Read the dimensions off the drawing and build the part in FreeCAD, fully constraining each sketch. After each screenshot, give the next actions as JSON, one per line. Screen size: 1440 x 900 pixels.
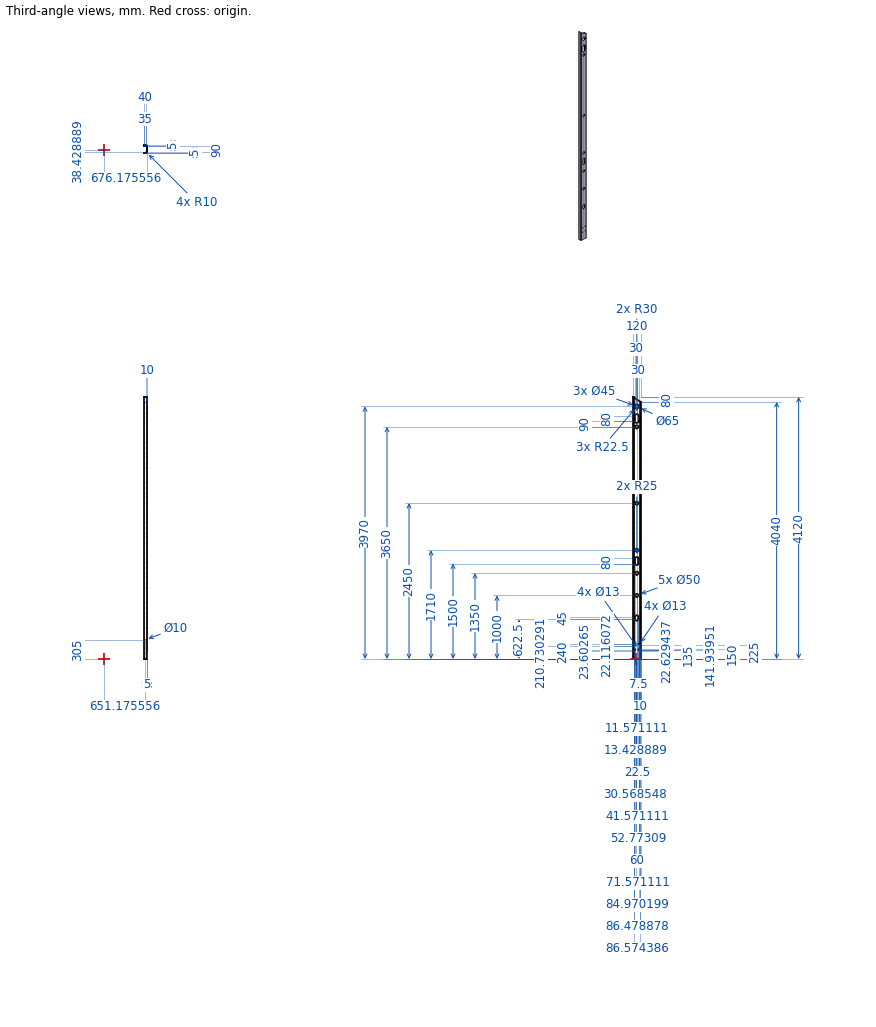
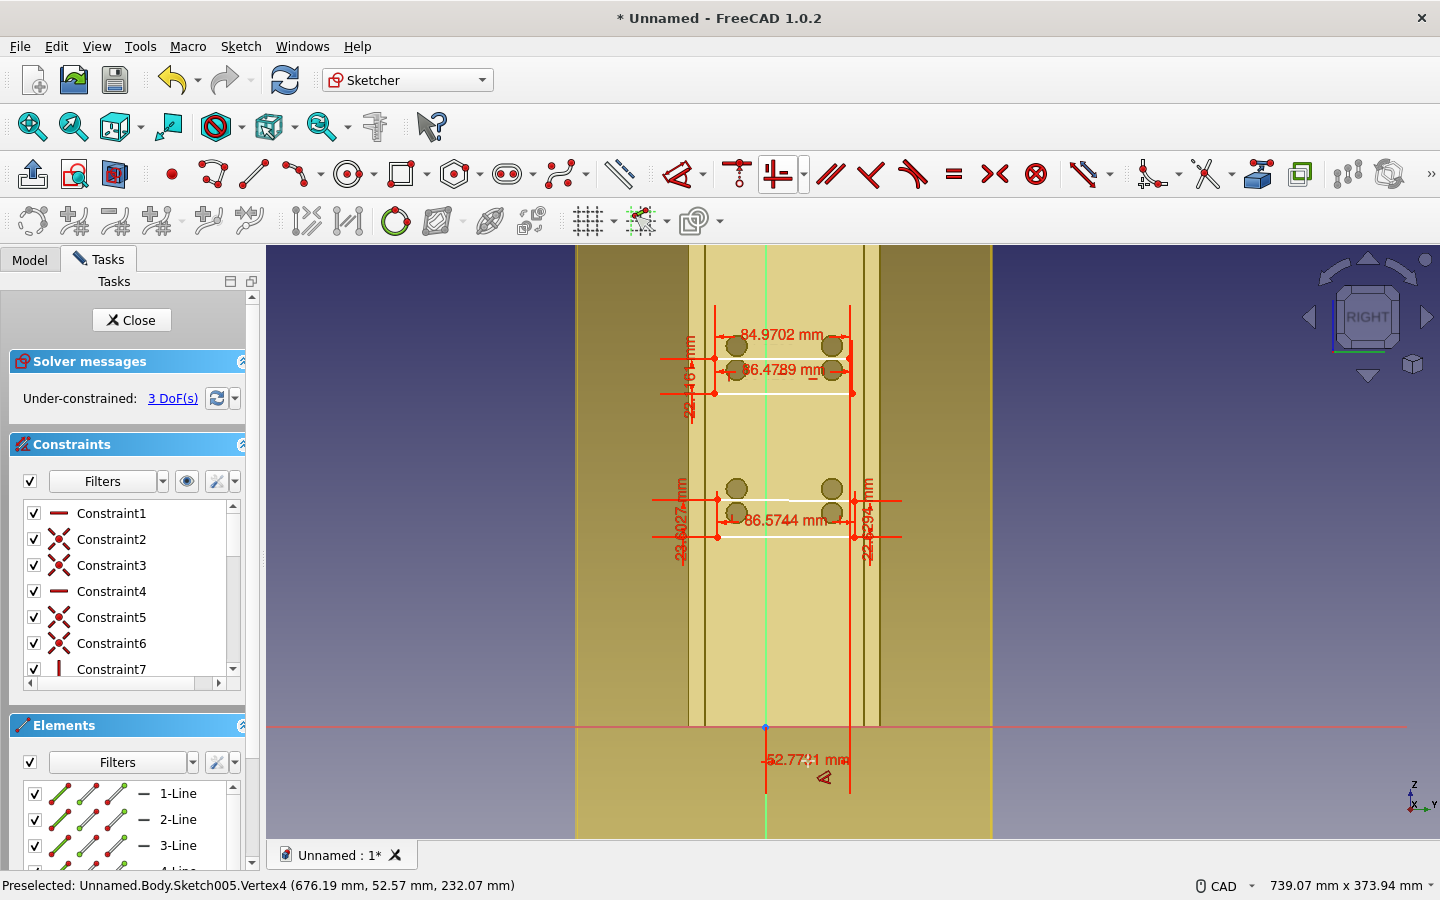
{"action": "left_click", "coordinate": [717, 537]}
{"action": "left_click", "coordinate": [730, 761]}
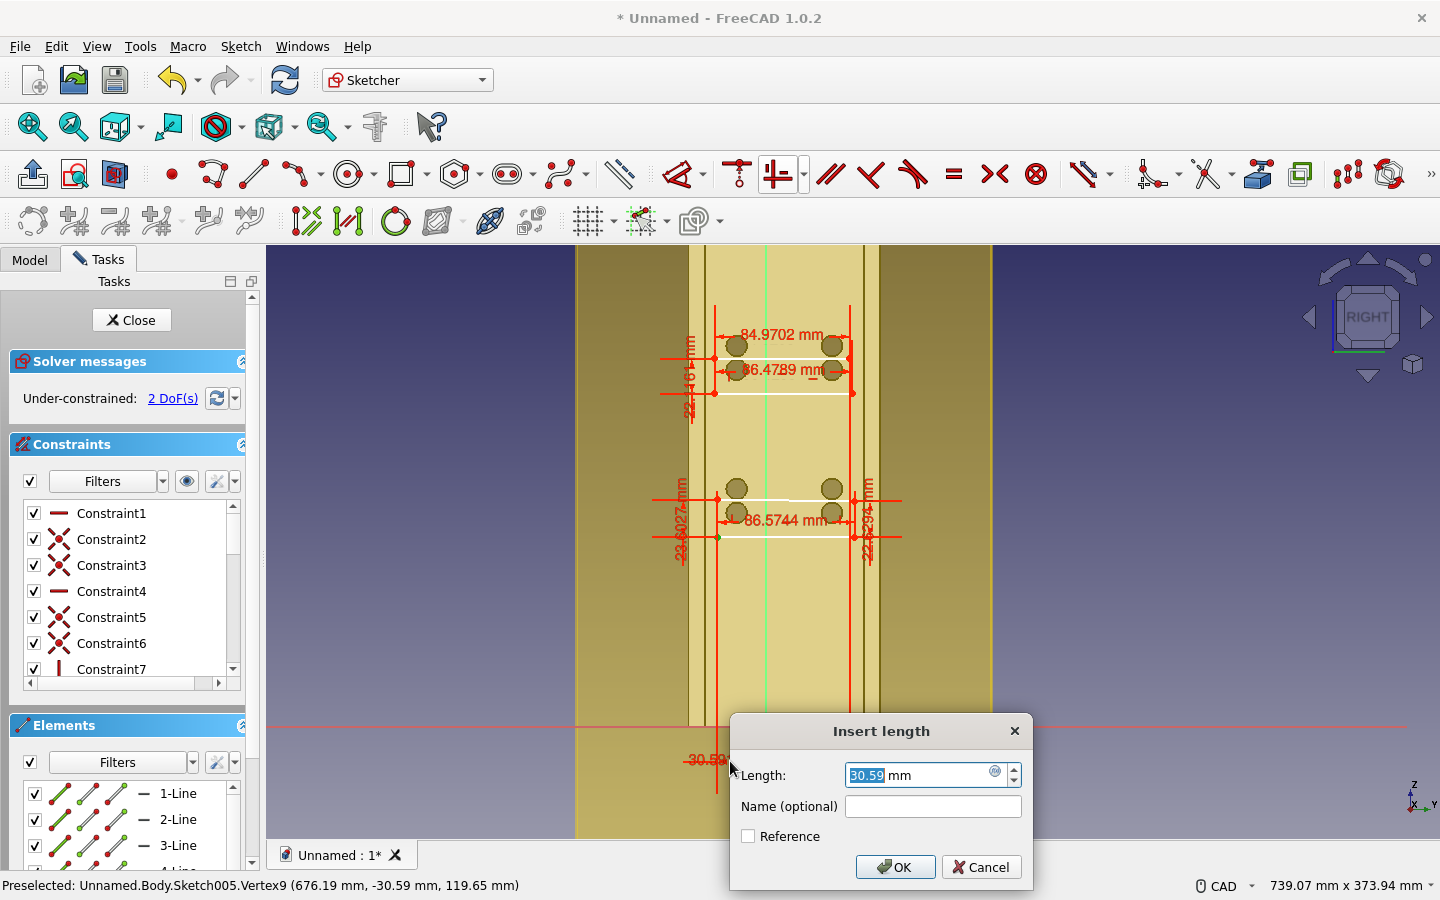
{"action": "type", "text": "30.568548"}
{"action": "key", "text": "Return"}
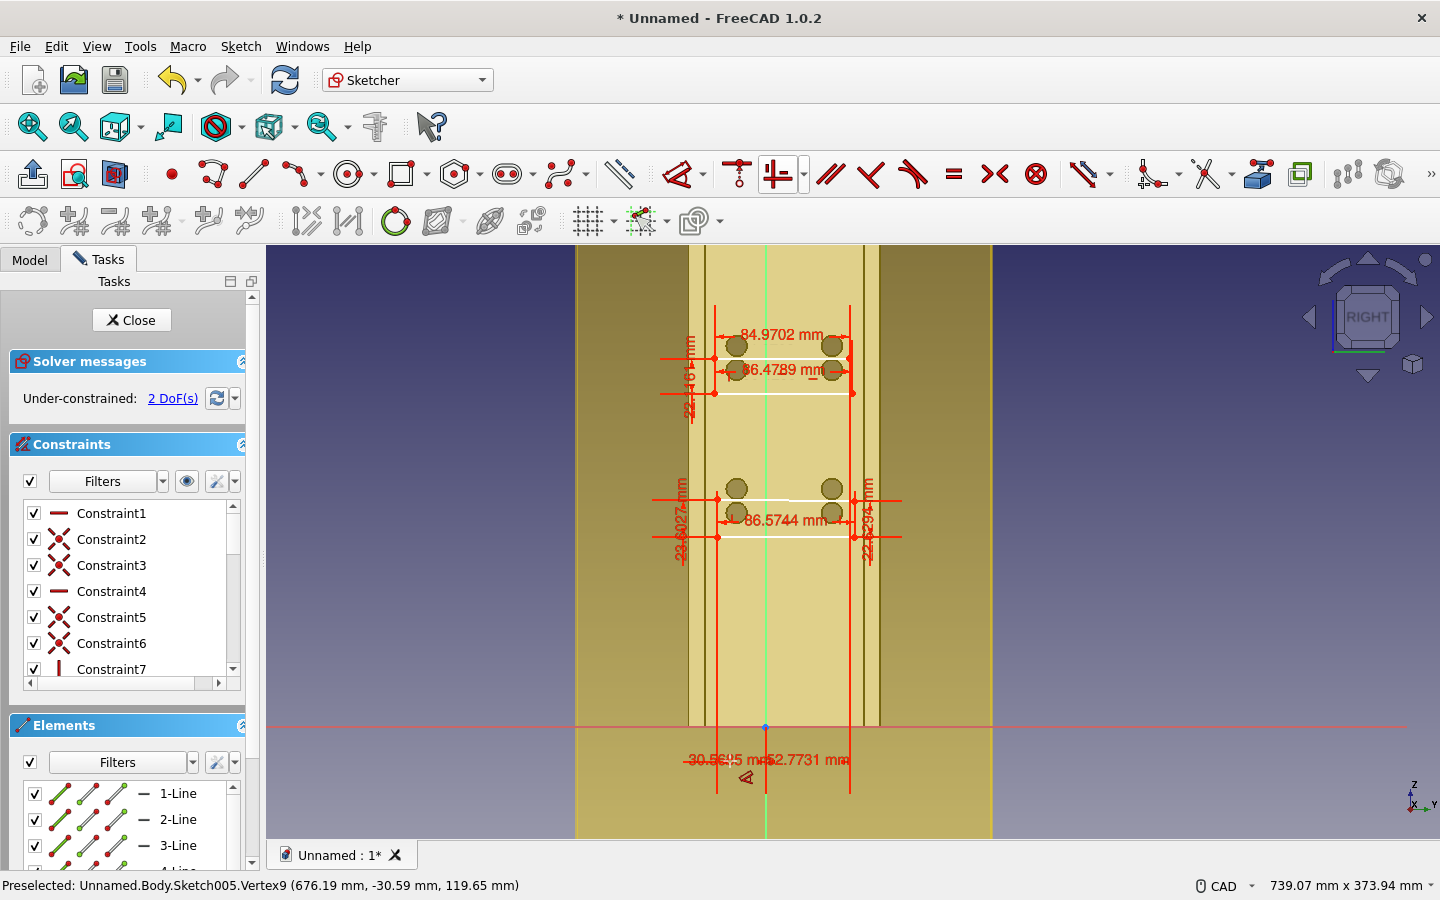
{"action": "left_click", "coordinate": [855, 501]}
{"action": "left_click", "coordinate": [889, 614]}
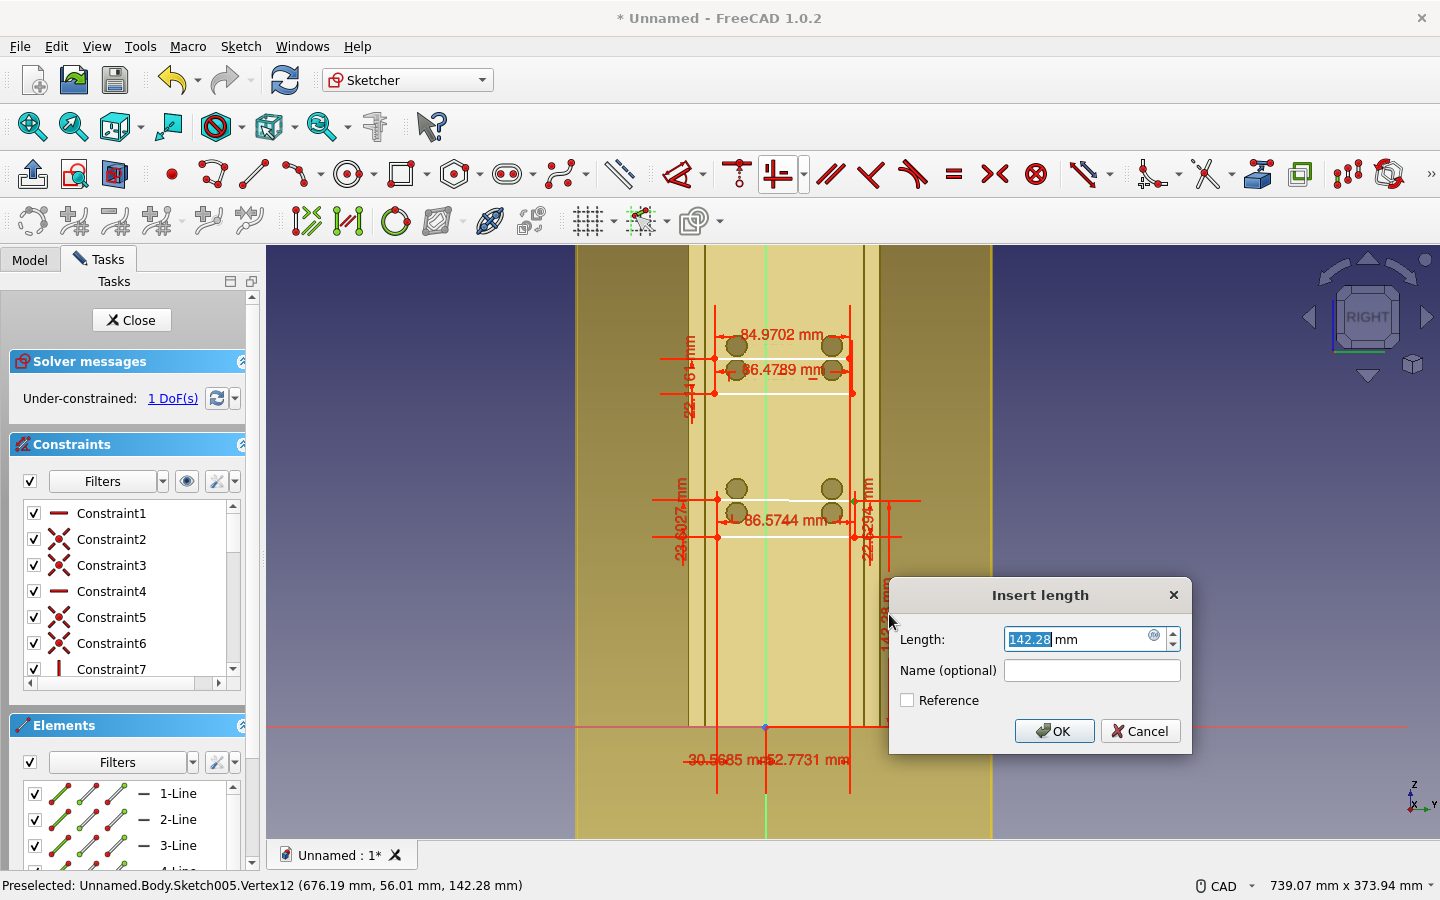
{"action": "type", "text": "141.93951"}
{"action": "key", "text": "Return"}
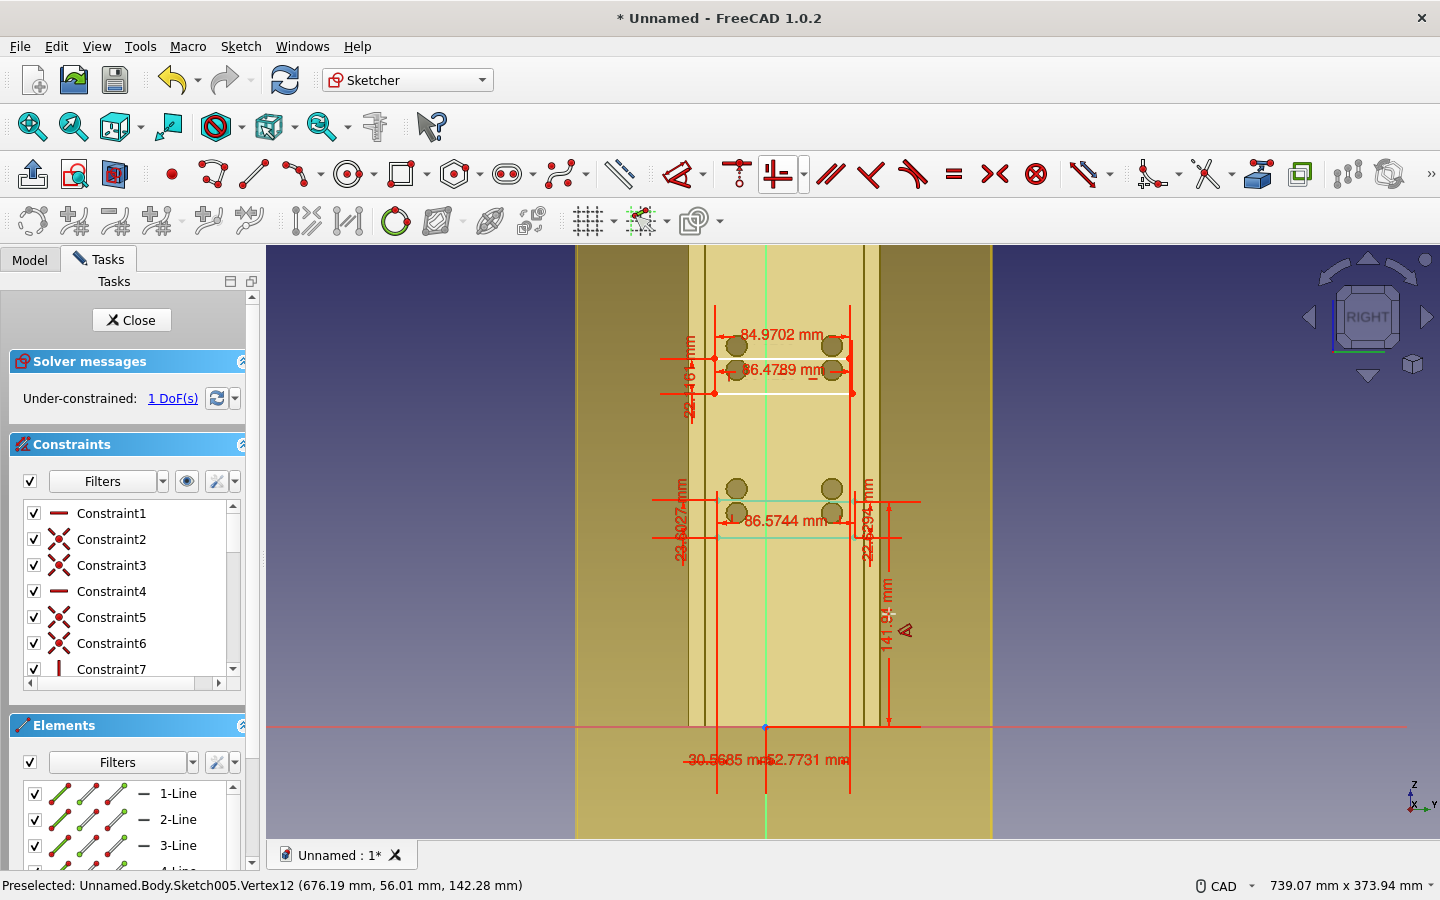
{"action": "left_click", "coordinate": [715, 394]}
{"action": "left_click", "coordinate": [681, 560]}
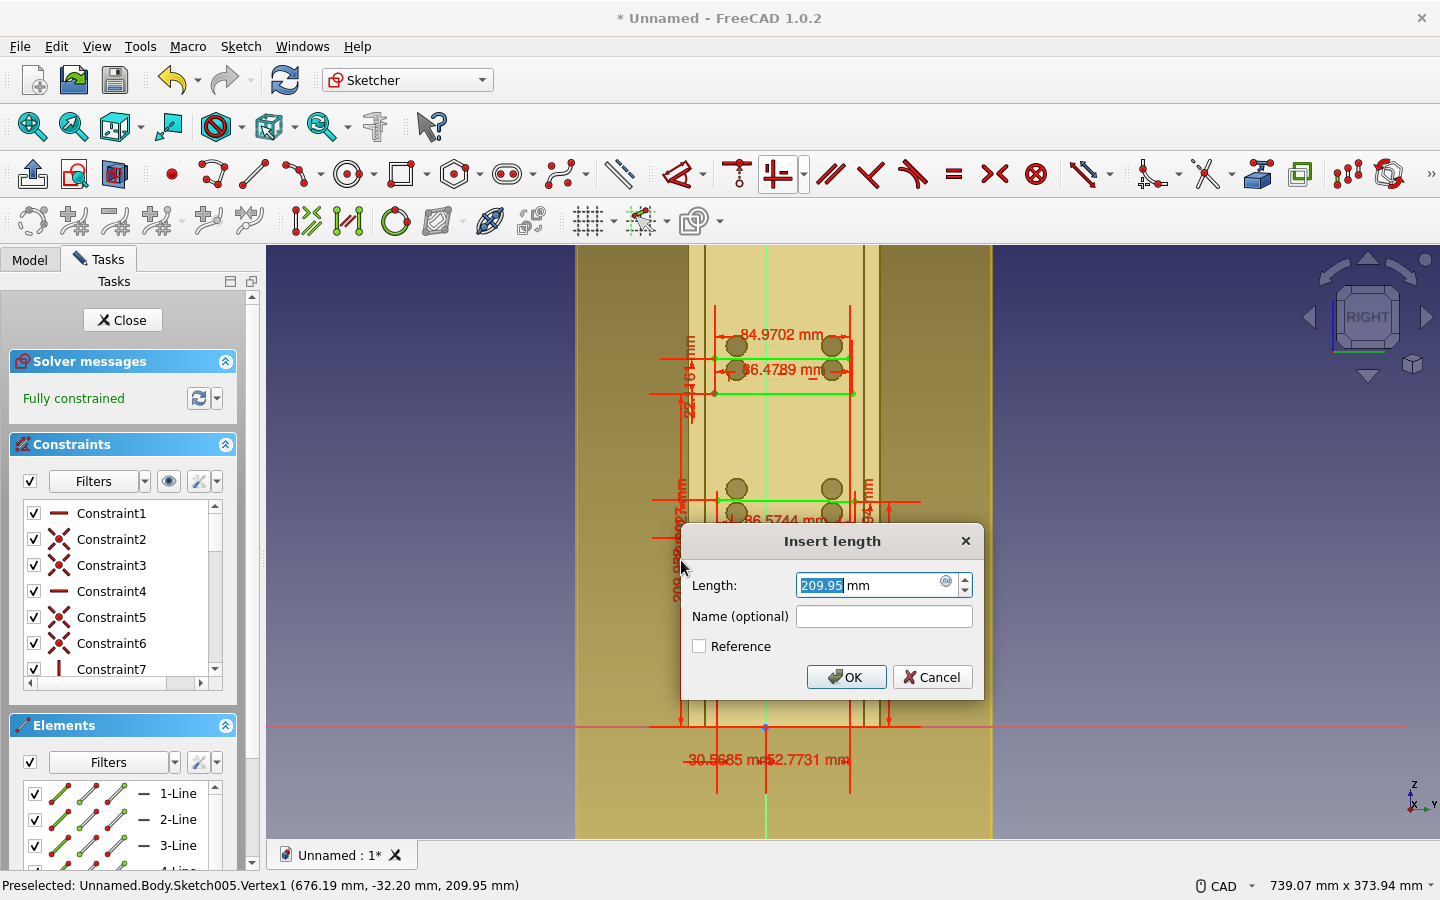
{"action": "type", "text": "210.730291"}
{"action": "key", "text": "Return"}
{"action": "key", "text": "Escape"}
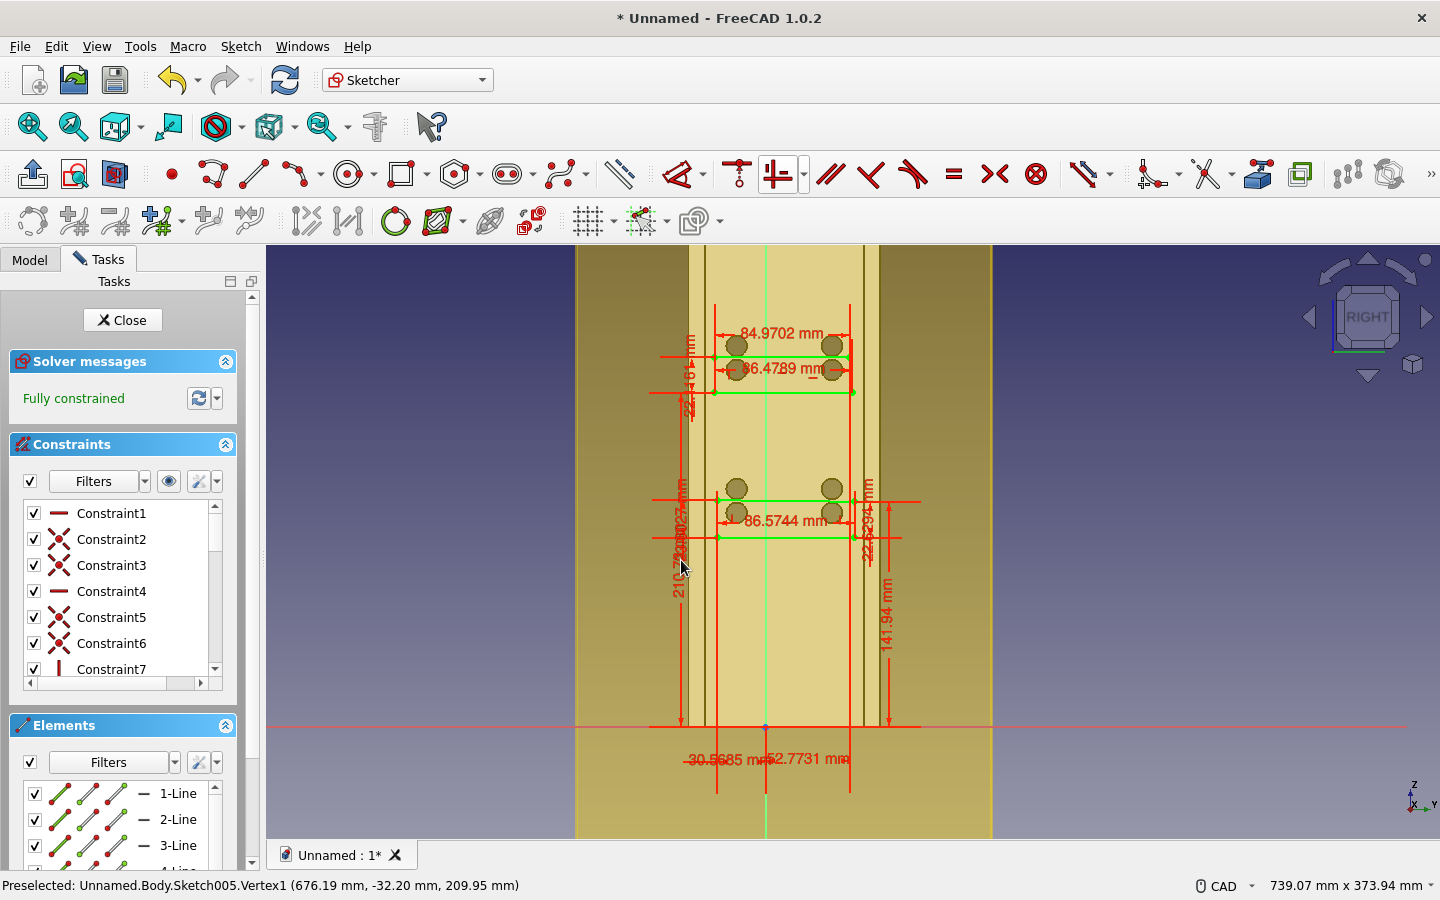
{"action": "left_click", "coordinate": [123, 320]}